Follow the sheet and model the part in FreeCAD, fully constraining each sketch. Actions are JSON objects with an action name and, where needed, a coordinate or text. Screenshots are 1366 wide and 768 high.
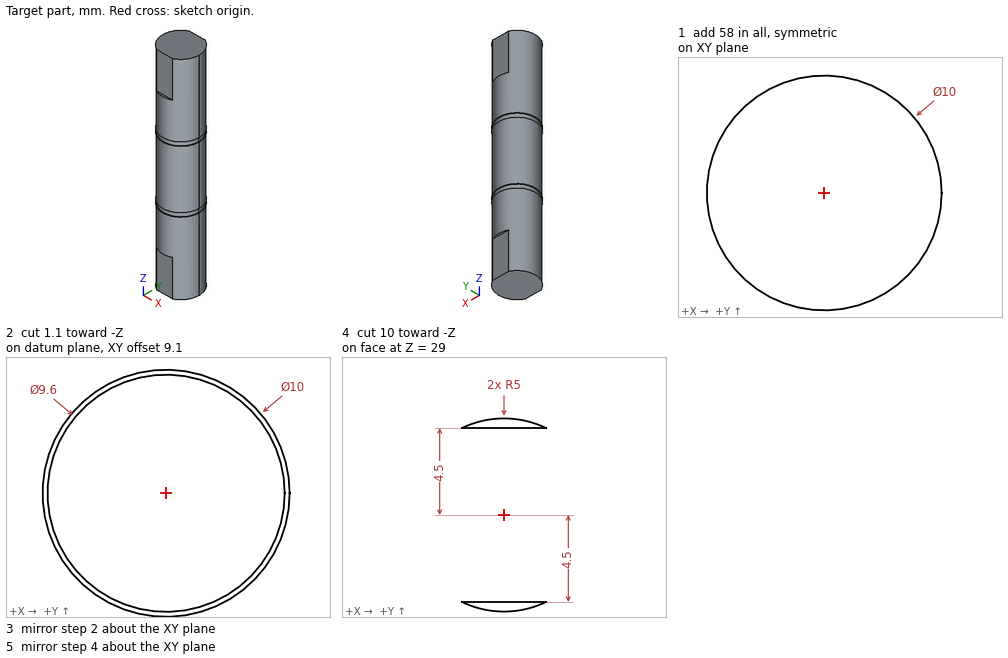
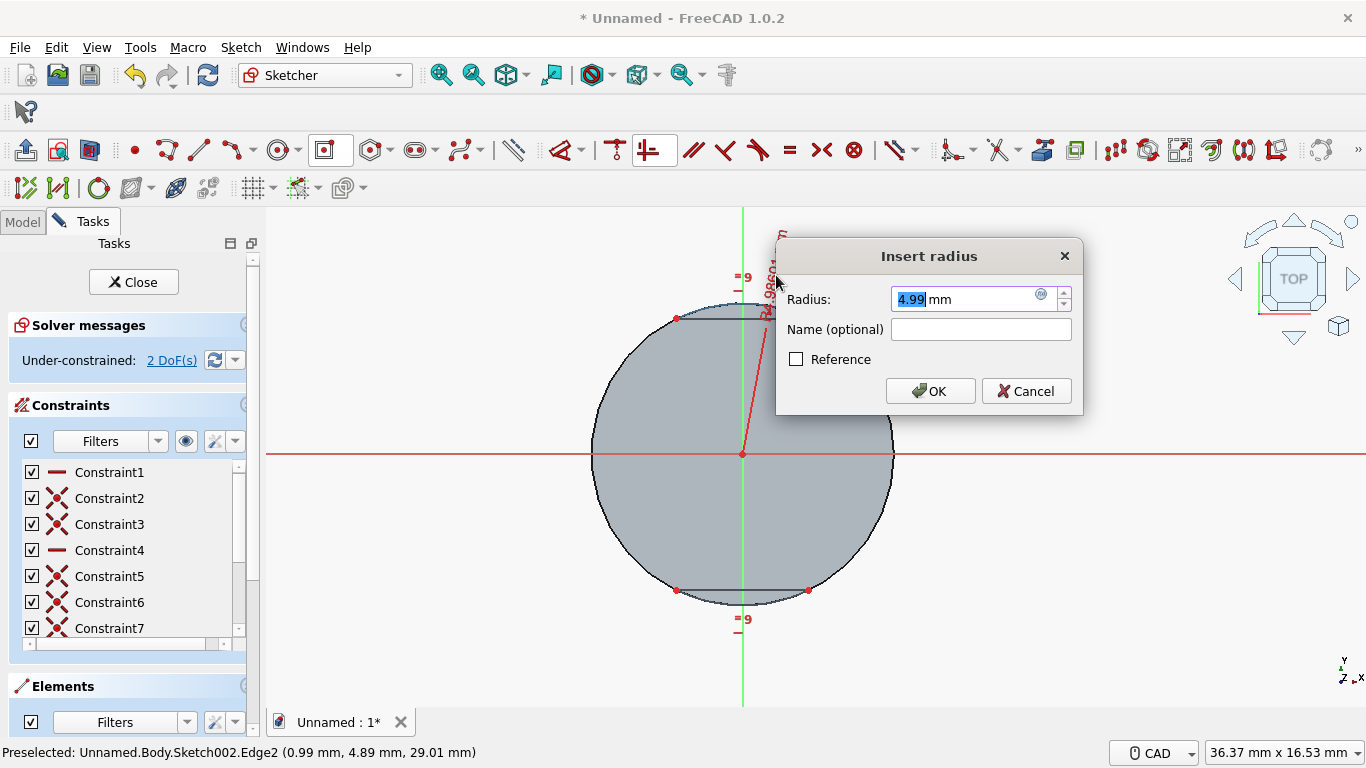
{"action": "type", "text": "5"}
{"action": "key", "text": "Return"}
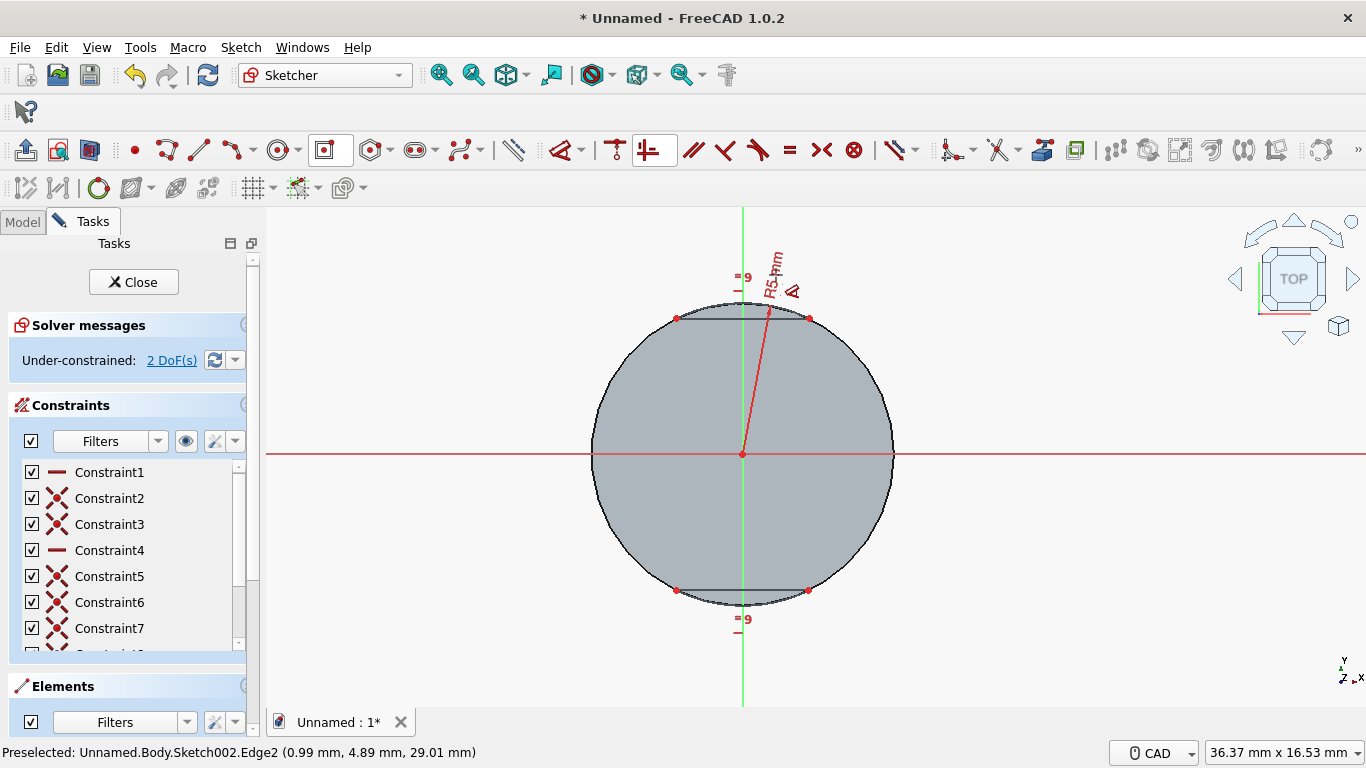
{"action": "left_click", "coordinate": [676, 319]}
{"action": "left_click", "coordinate": [642, 386]}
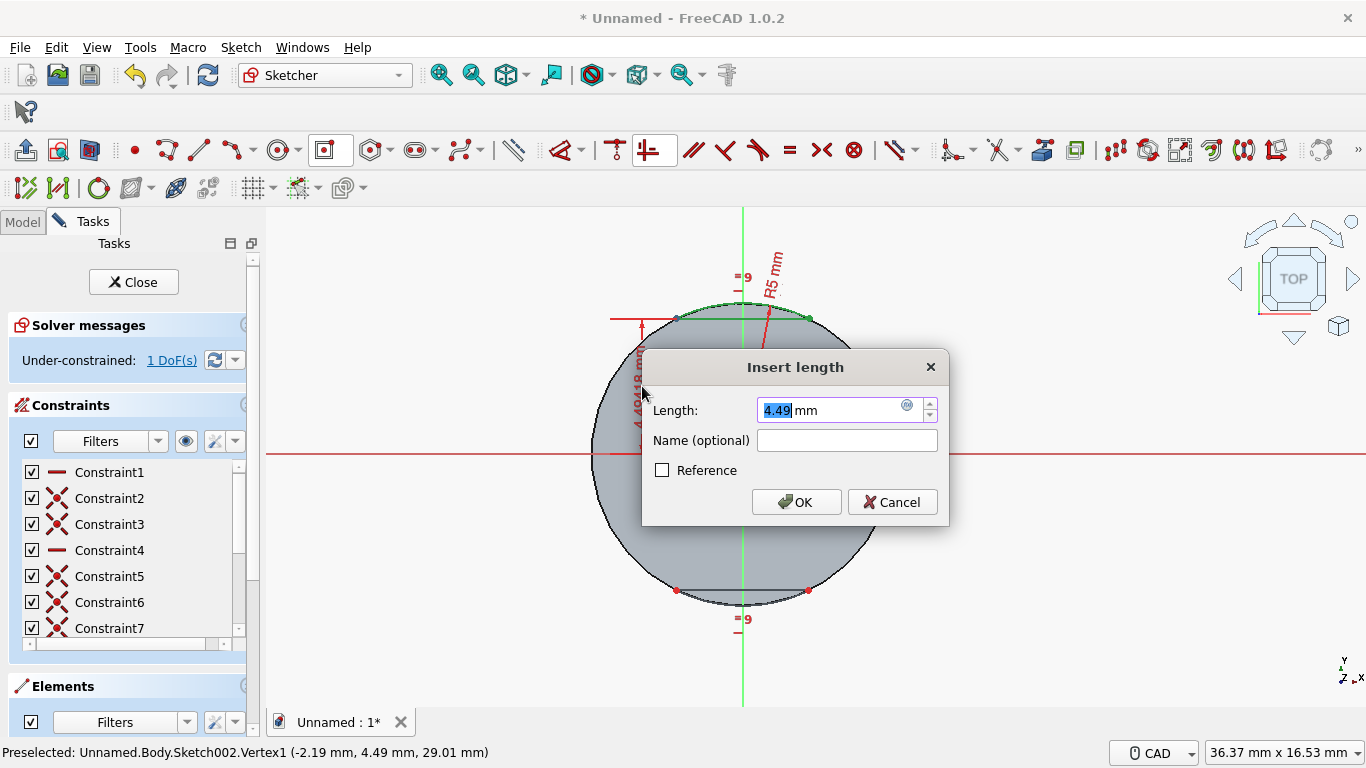
{"action": "type", "text": "4.5"}
{"action": "key", "text": "Return"}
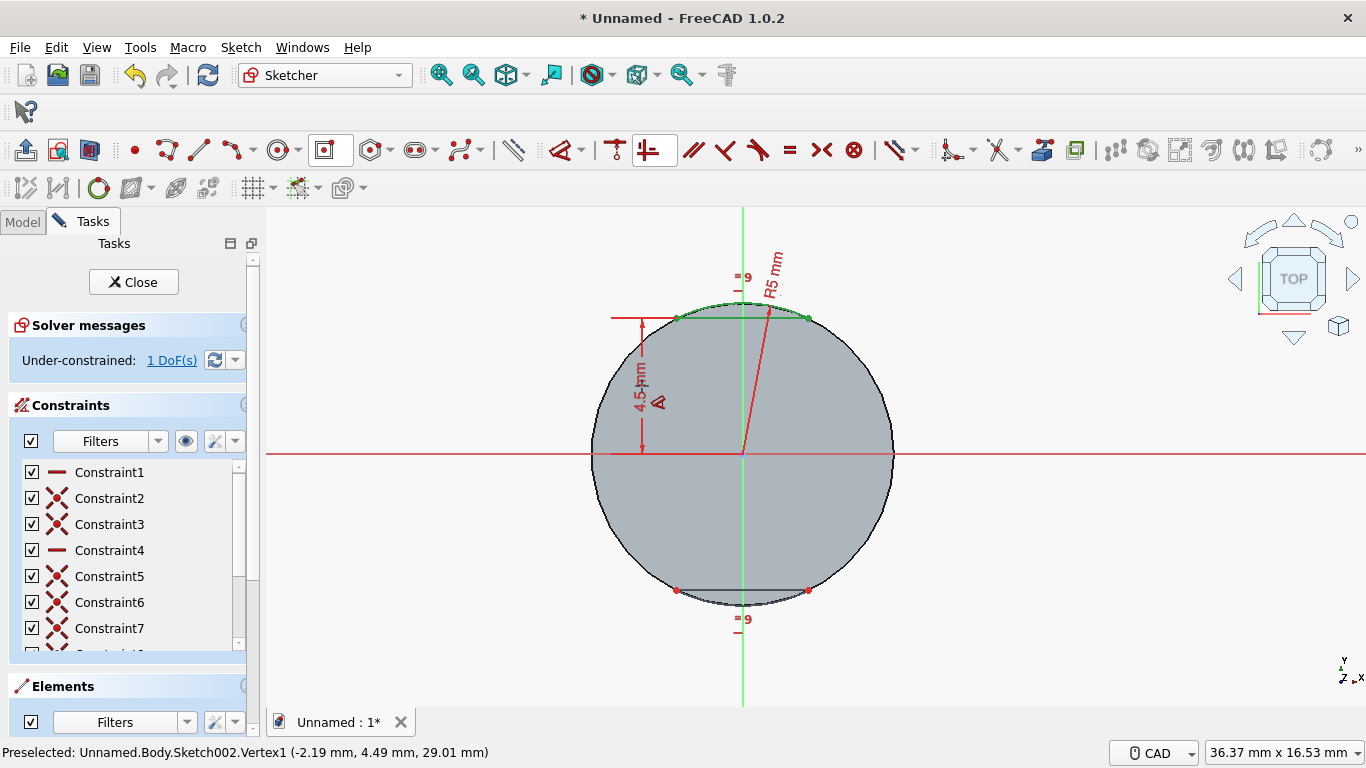
{"action": "left_click", "coordinate": [809, 590]}
{"action": "left_click", "coordinate": [843, 522]}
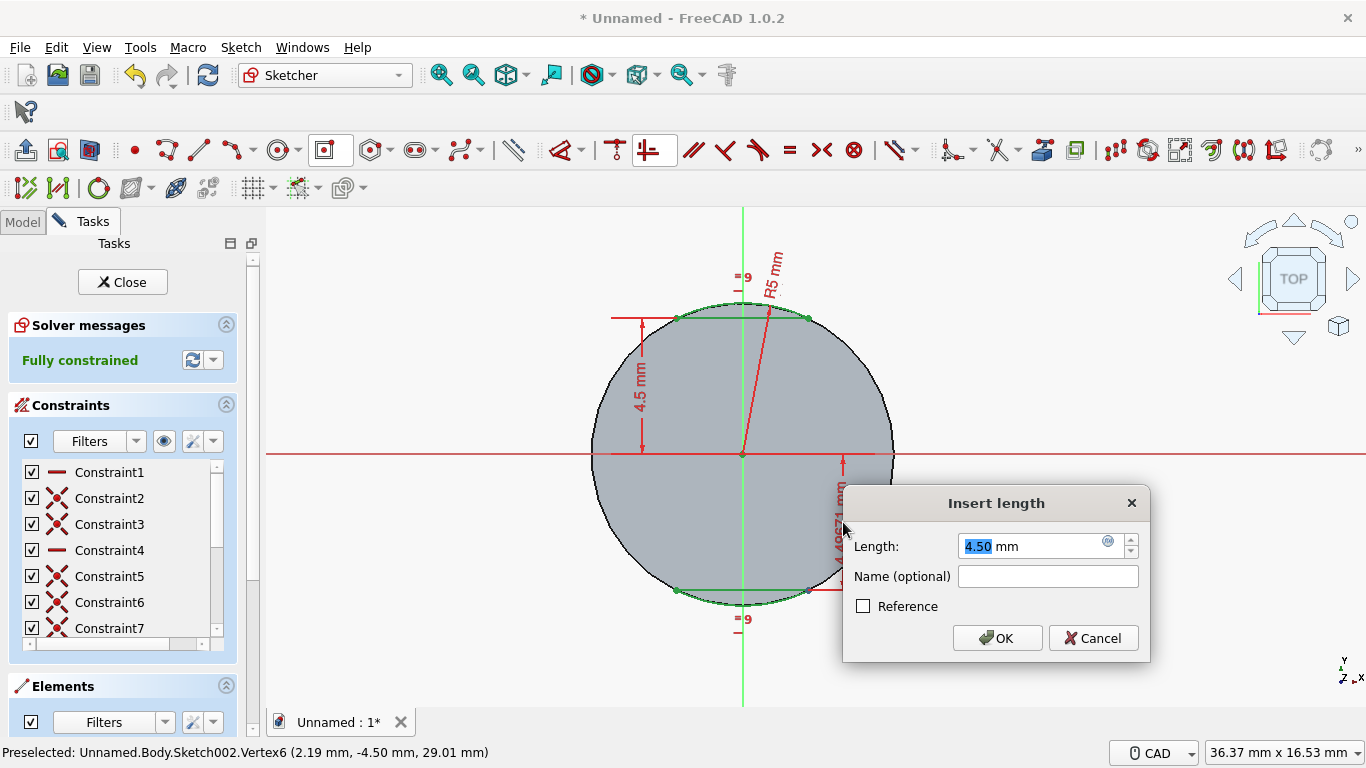
{"action": "type", "text": "4.5"}
{"action": "key", "text": "Return"}
{"action": "key", "text": "Escape"}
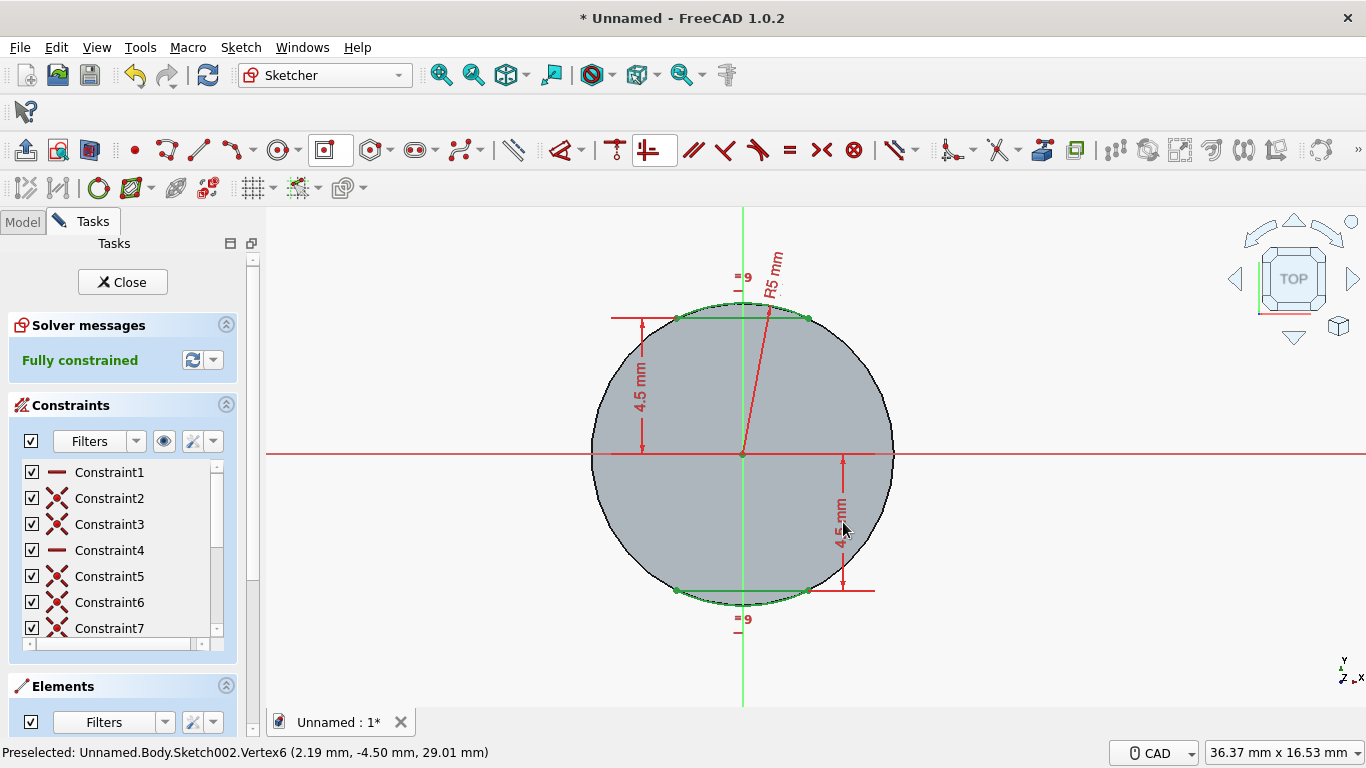
{"action": "left_click", "coordinate": [123, 282]}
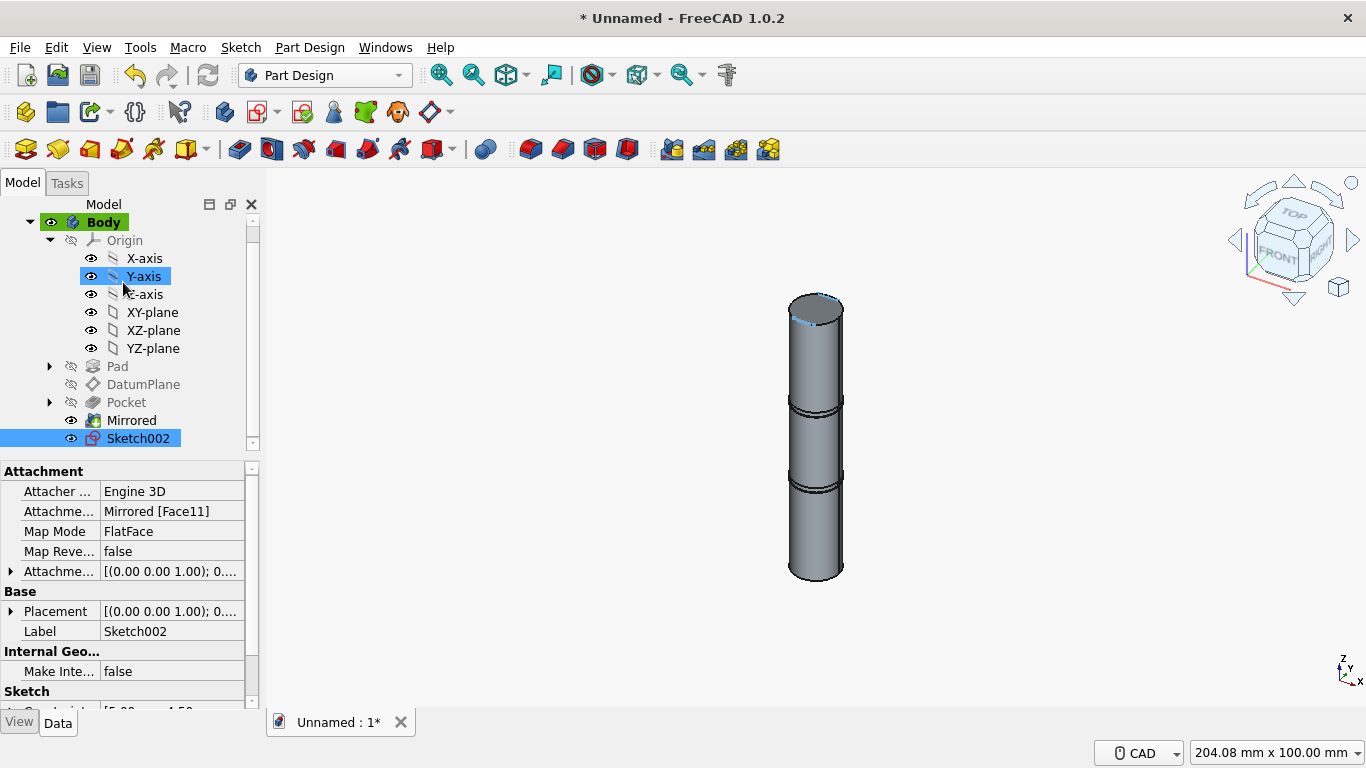
{"action": "left_click", "coordinate": [240, 150]}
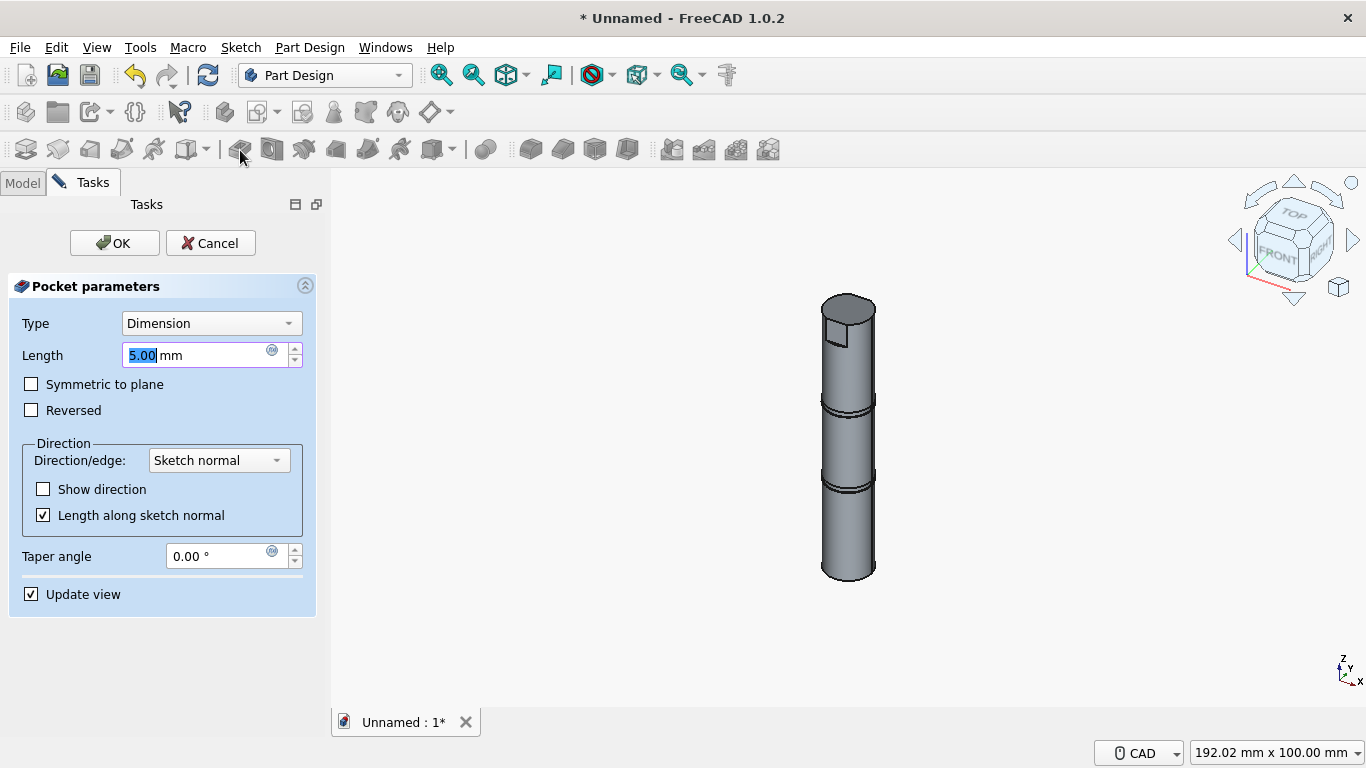
{"action": "type", "text": "10"}
{"action": "key", "text": "Tab"}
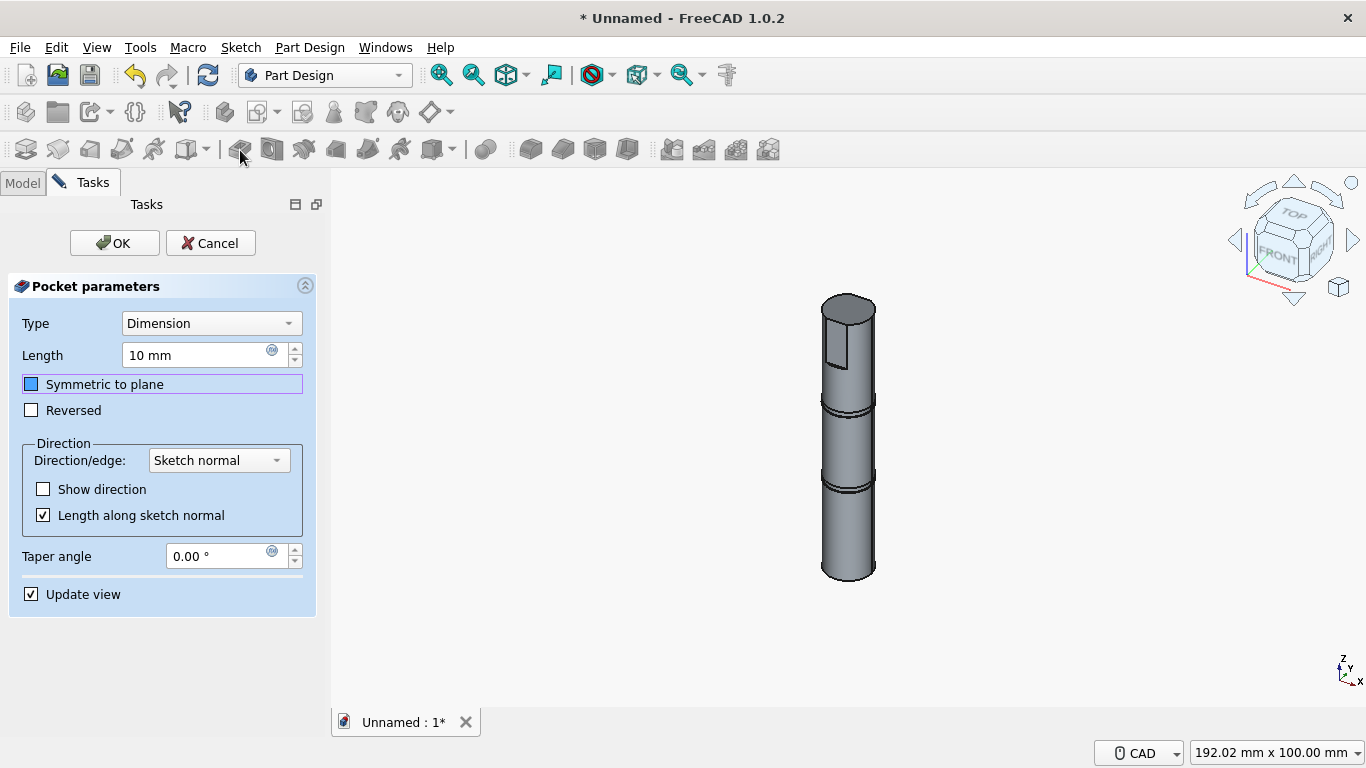
{"action": "left_click", "coordinate": [115, 243]}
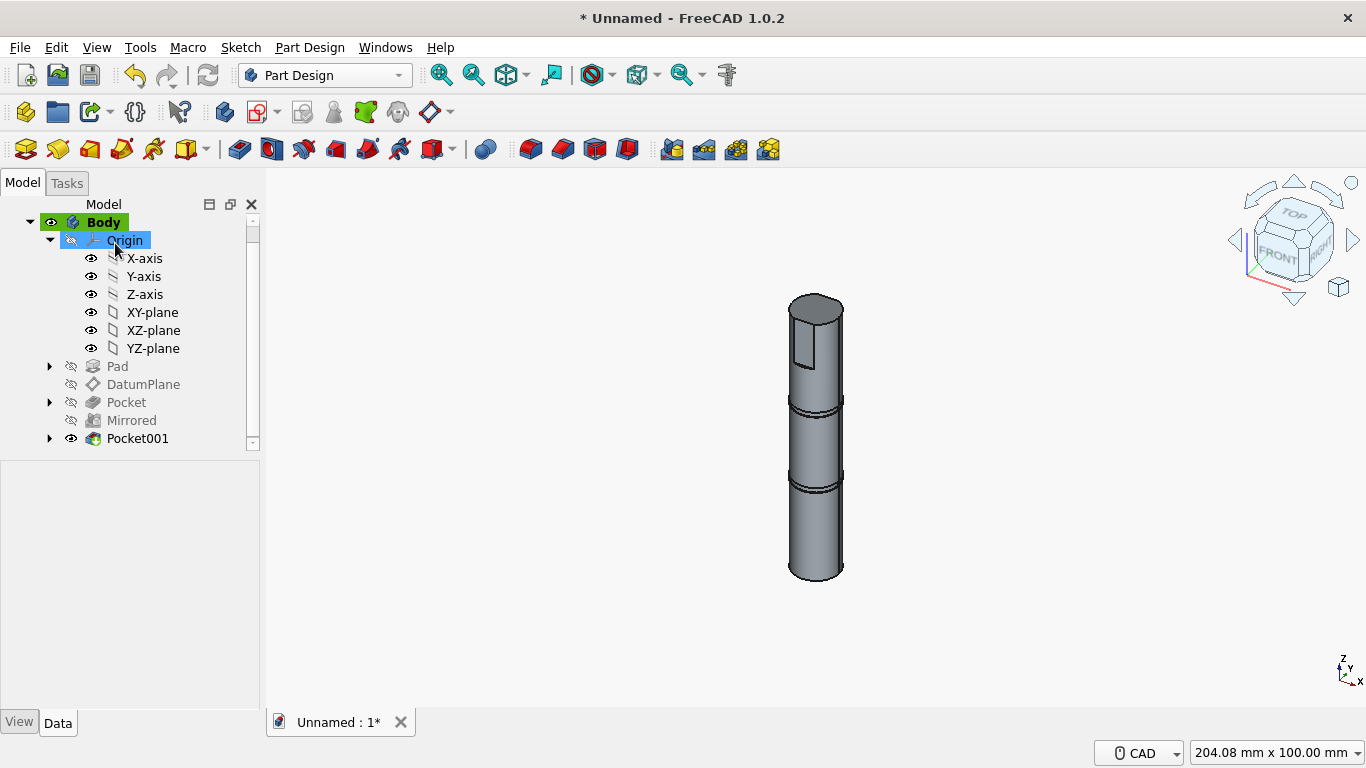
{"action": "left_click", "coordinate": [116, 438]}